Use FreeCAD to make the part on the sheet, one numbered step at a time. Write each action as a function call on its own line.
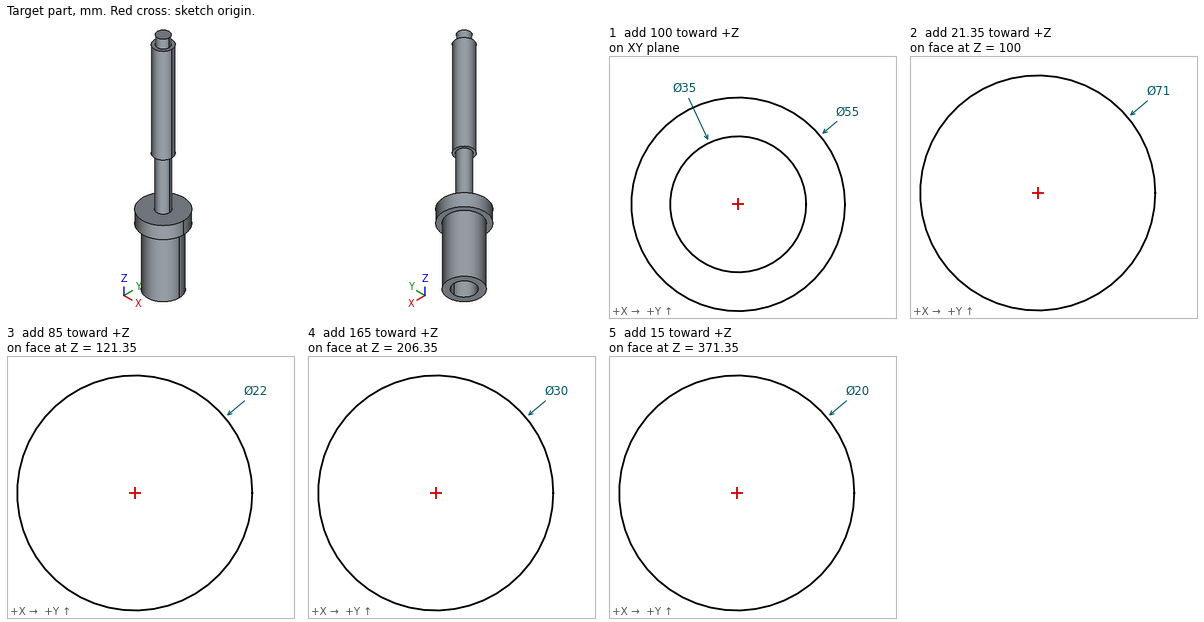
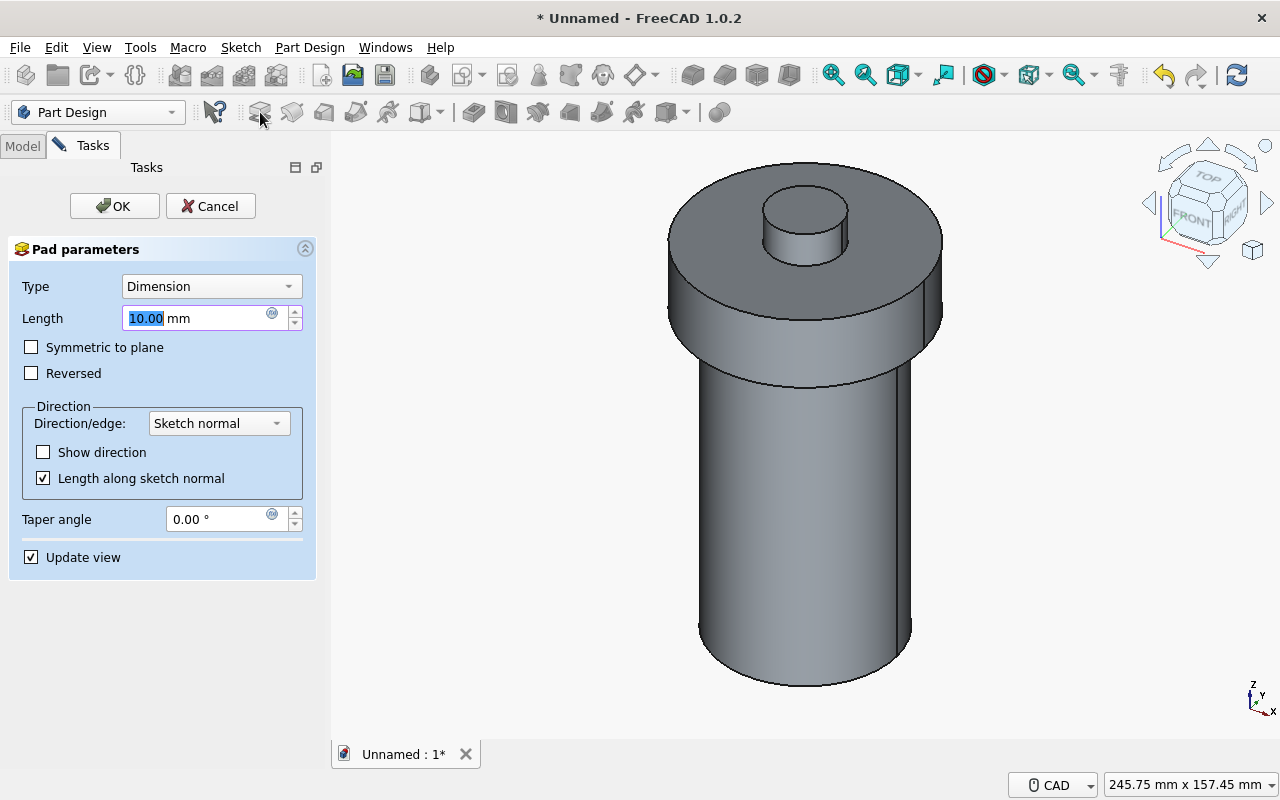
text(85)
key(Tab)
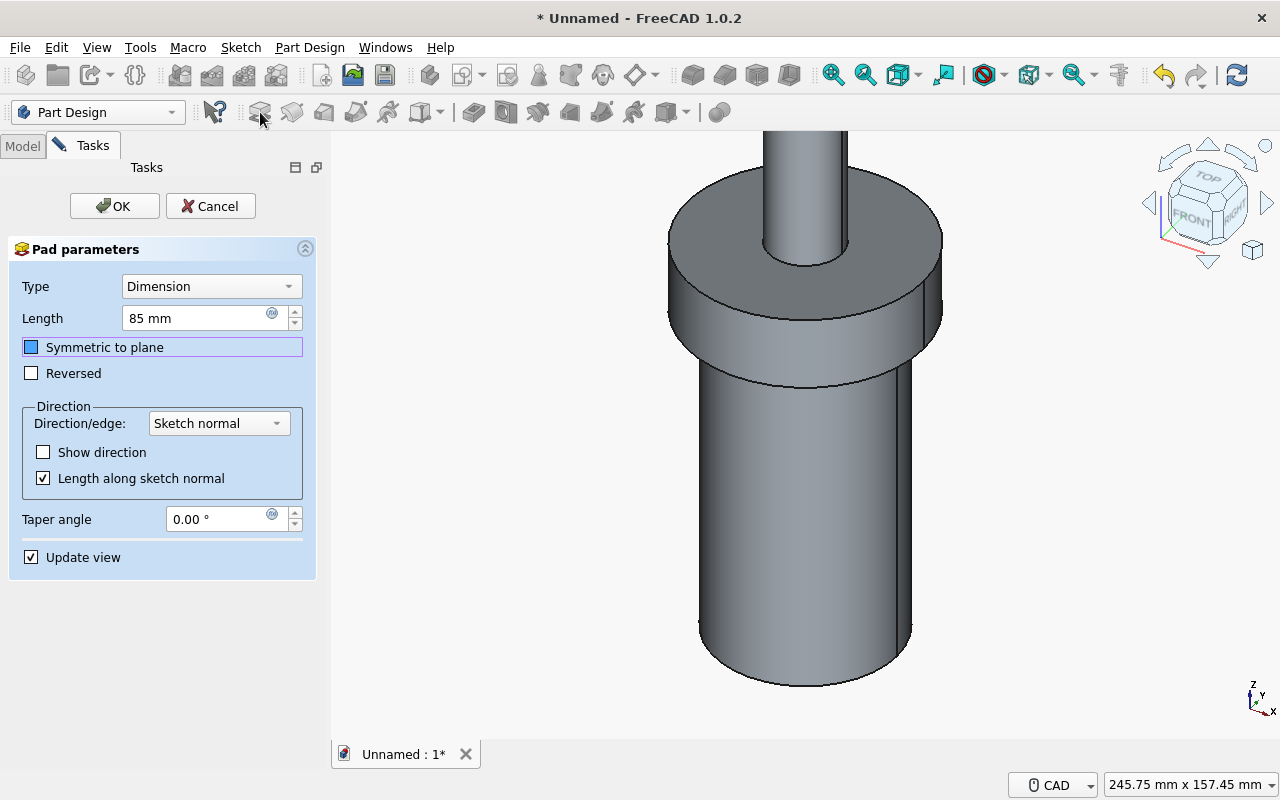
click(115, 206)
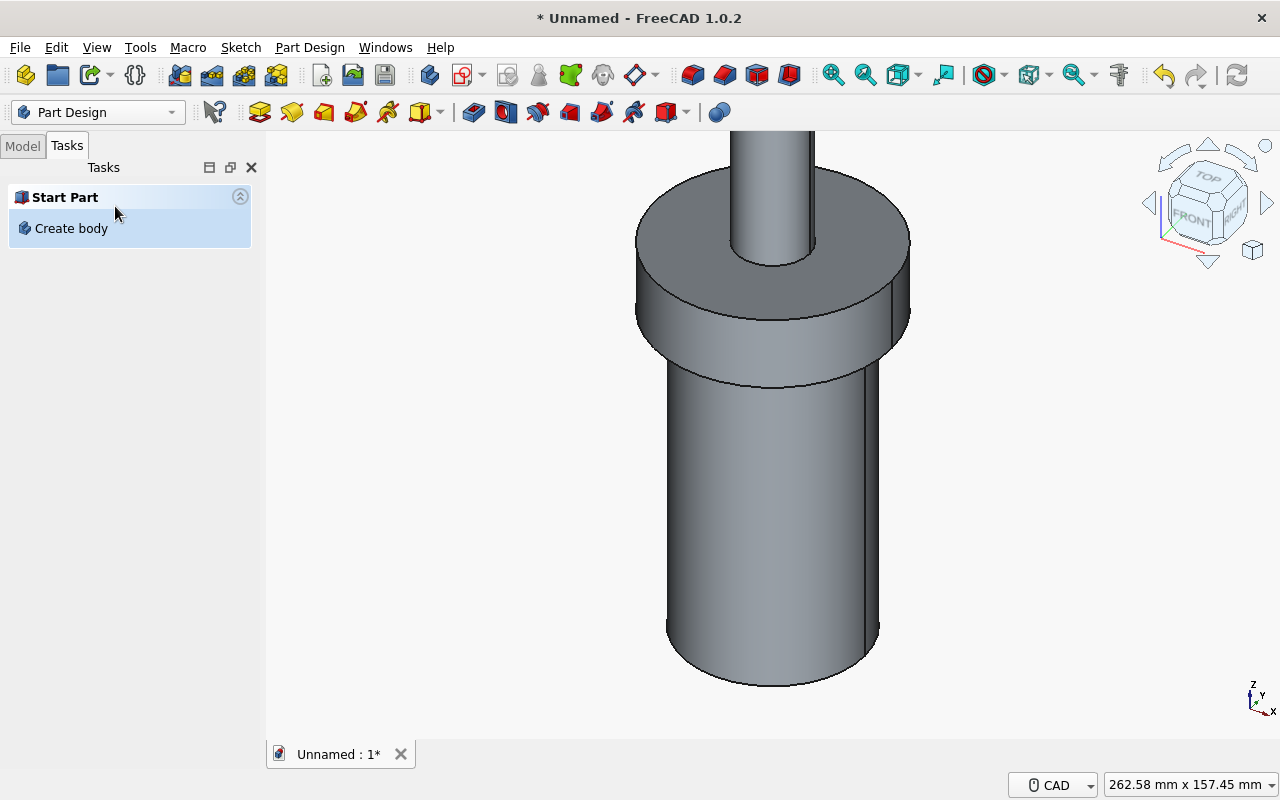
key(v)
key(f)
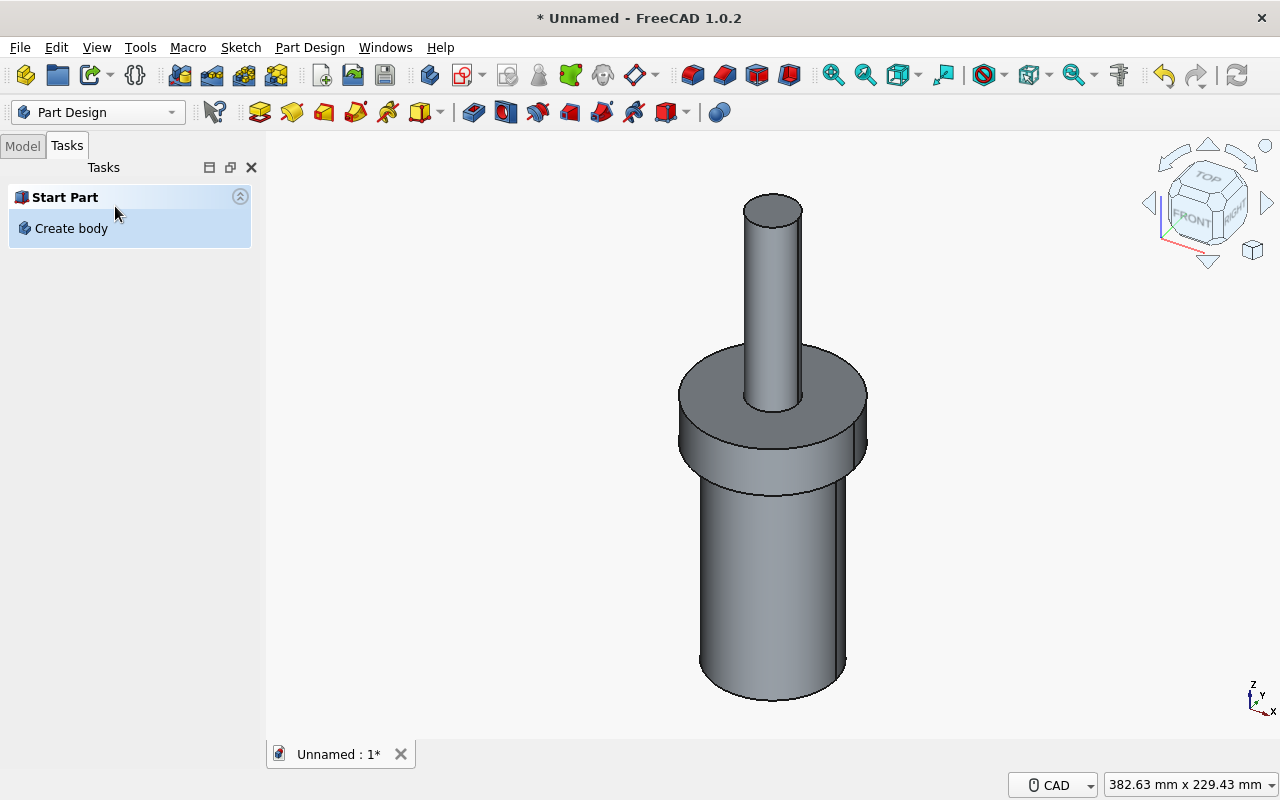
click(773, 210)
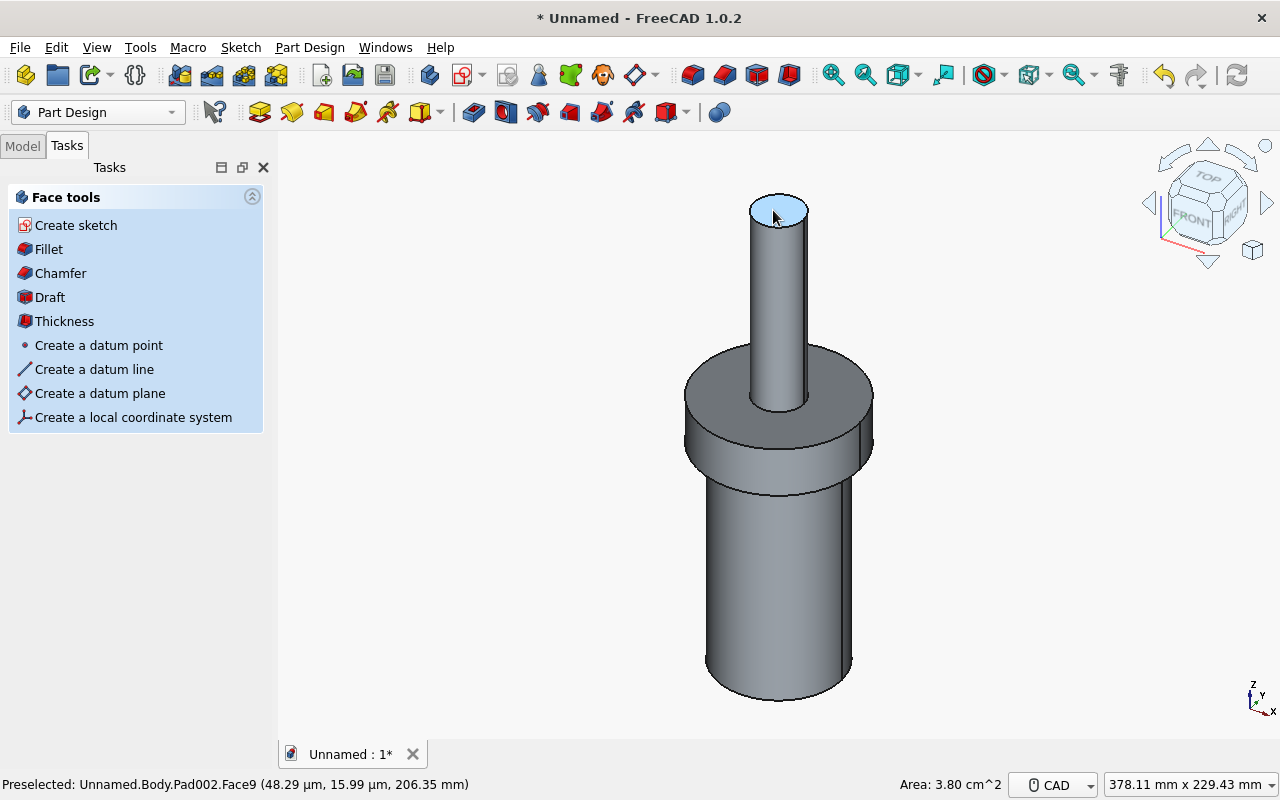
click(462, 76)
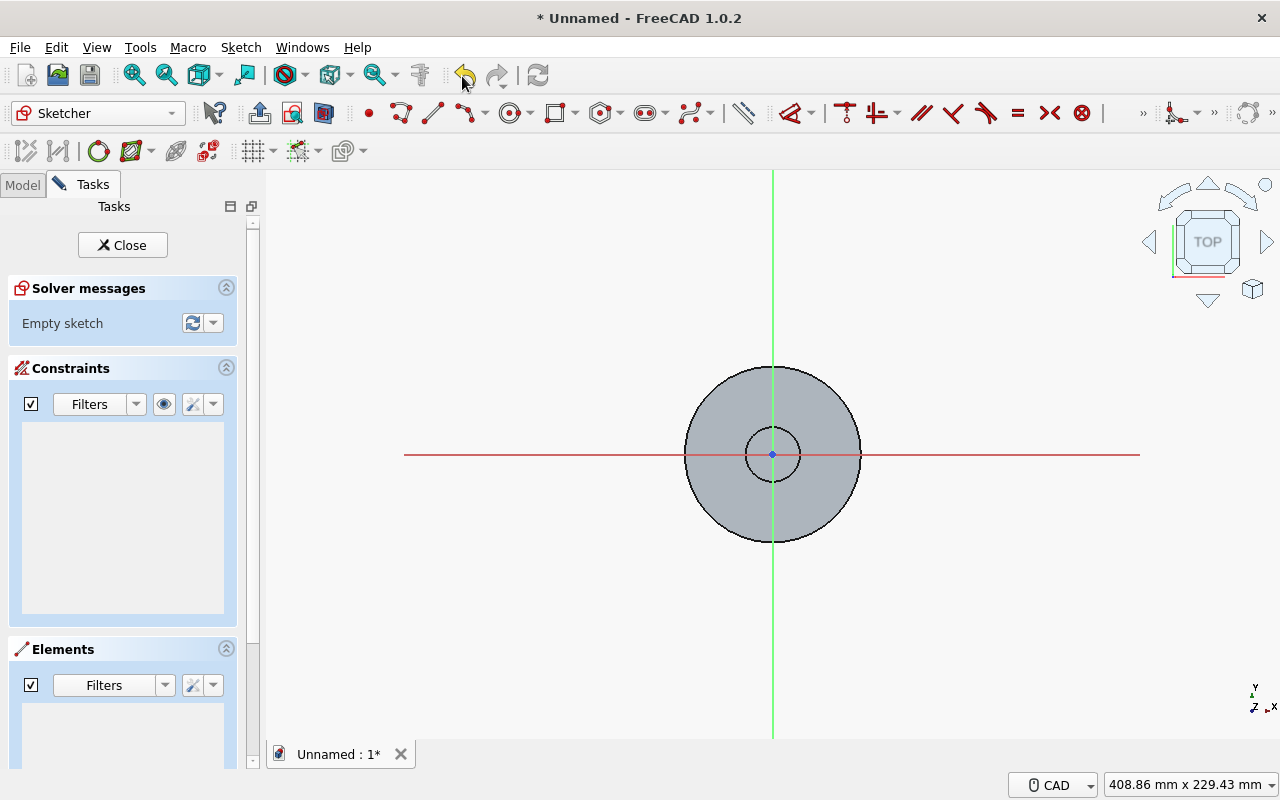
scroll(790, 454, up, 8)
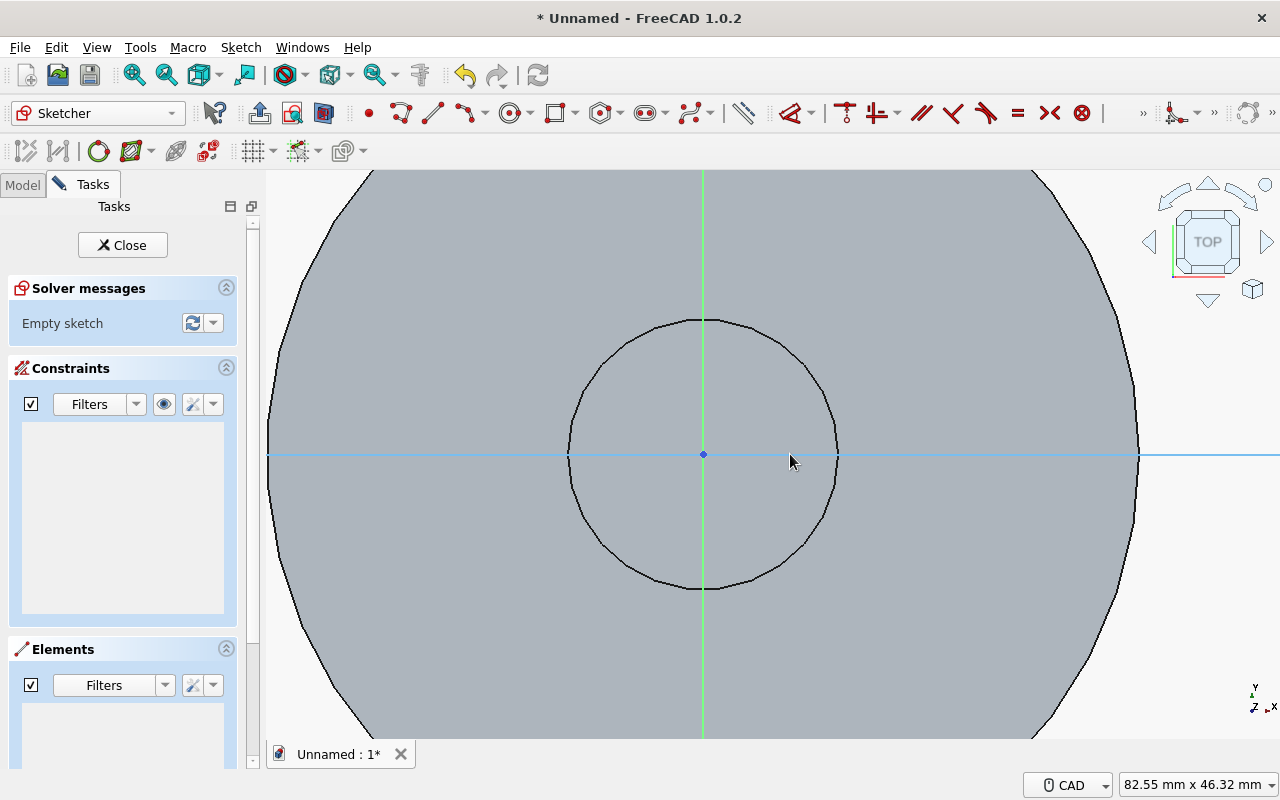
key(g)
key(c)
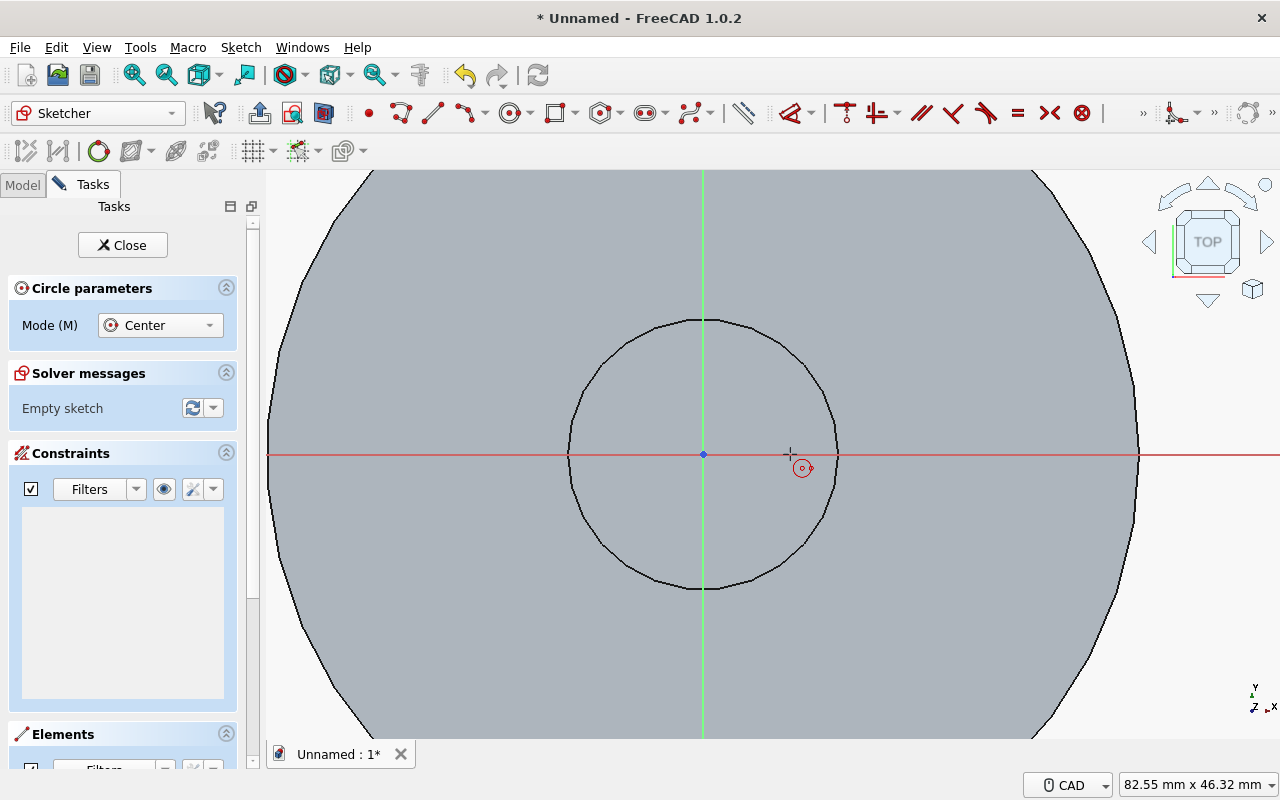
click(703, 454)
click(833, 324)
key(Escape)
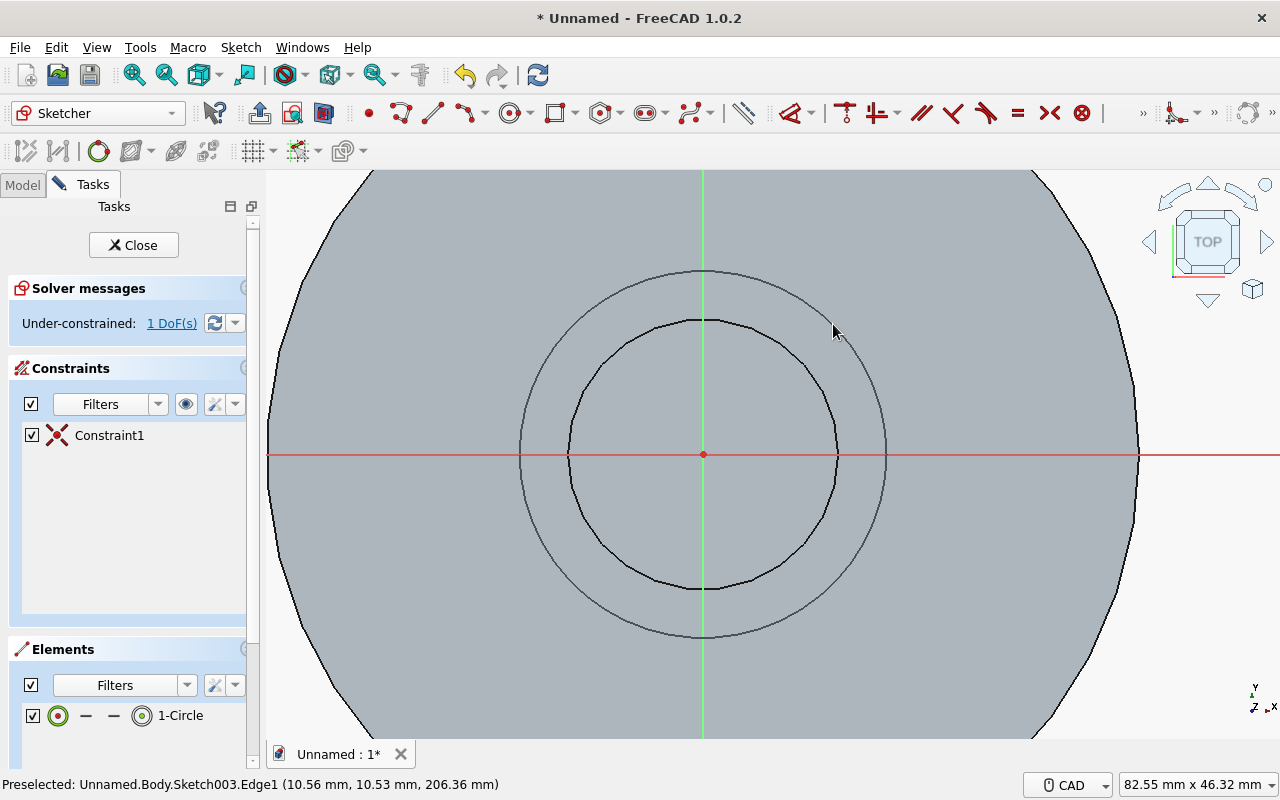
click(832, 324)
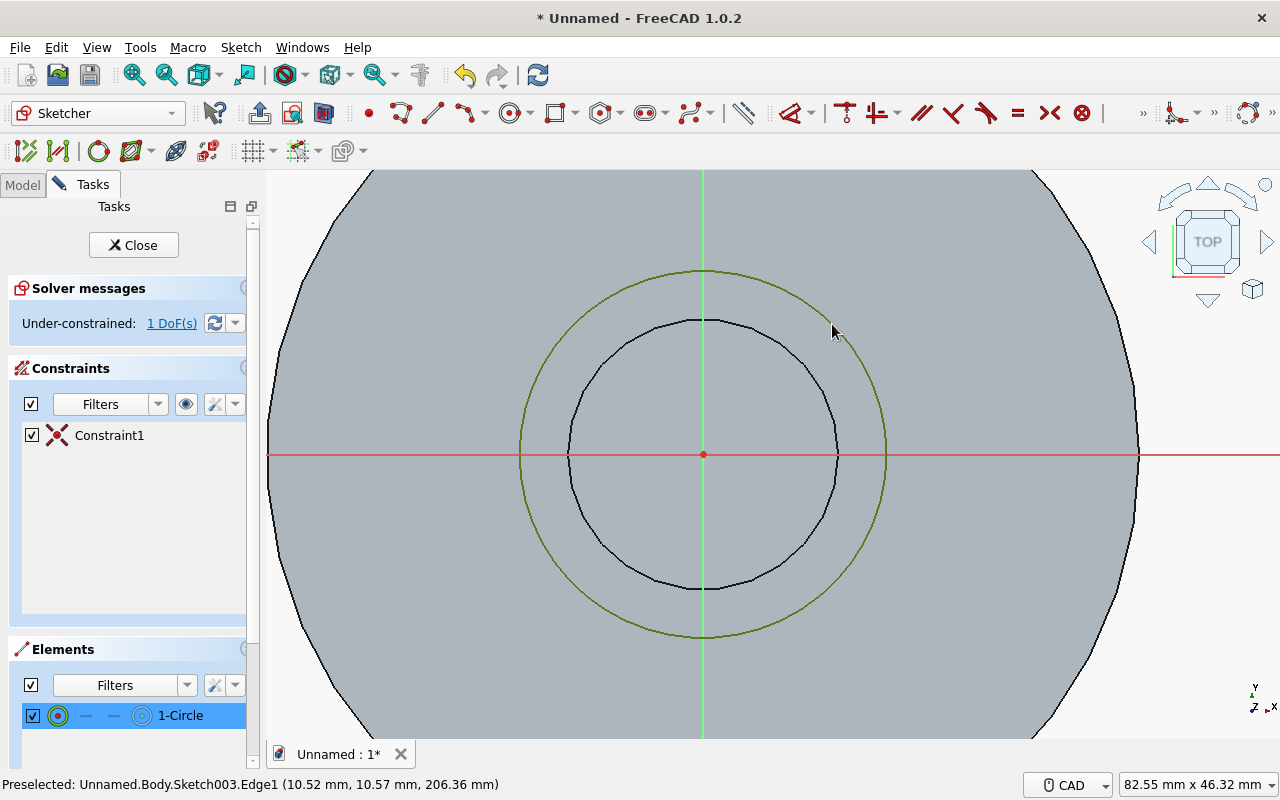
key(k)
key(o)